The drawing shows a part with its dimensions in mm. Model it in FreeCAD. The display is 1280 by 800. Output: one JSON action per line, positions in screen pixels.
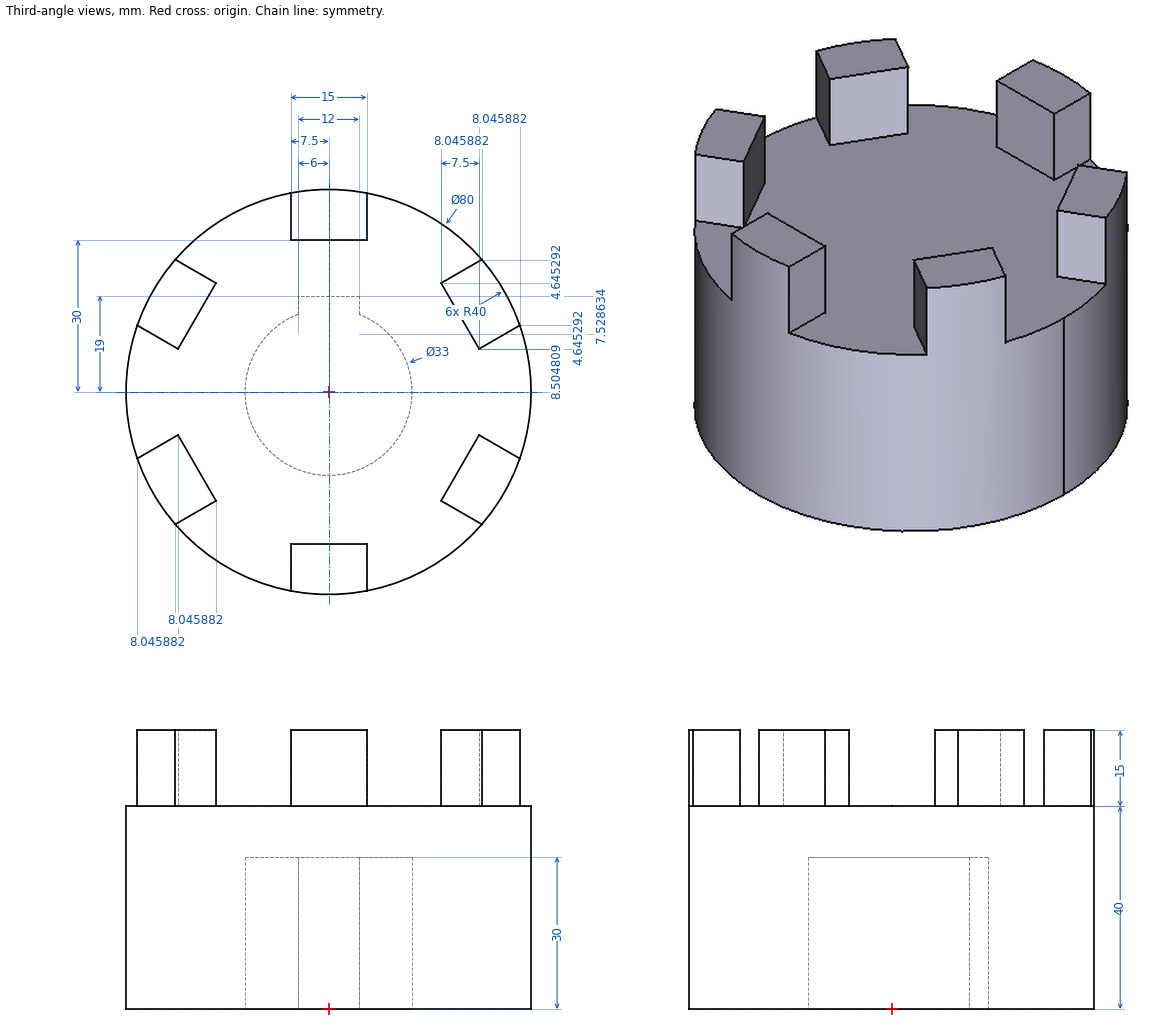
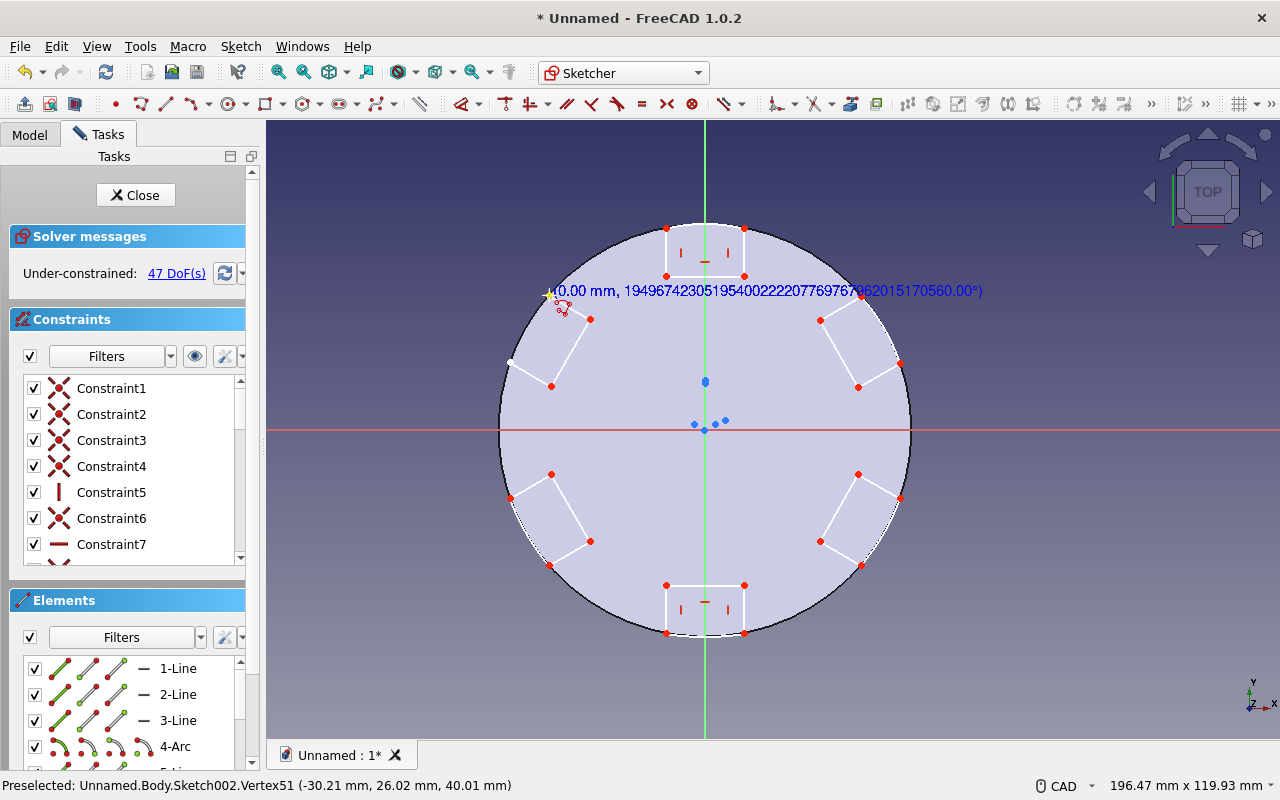
{"action": "key", "text": "g 3 a"}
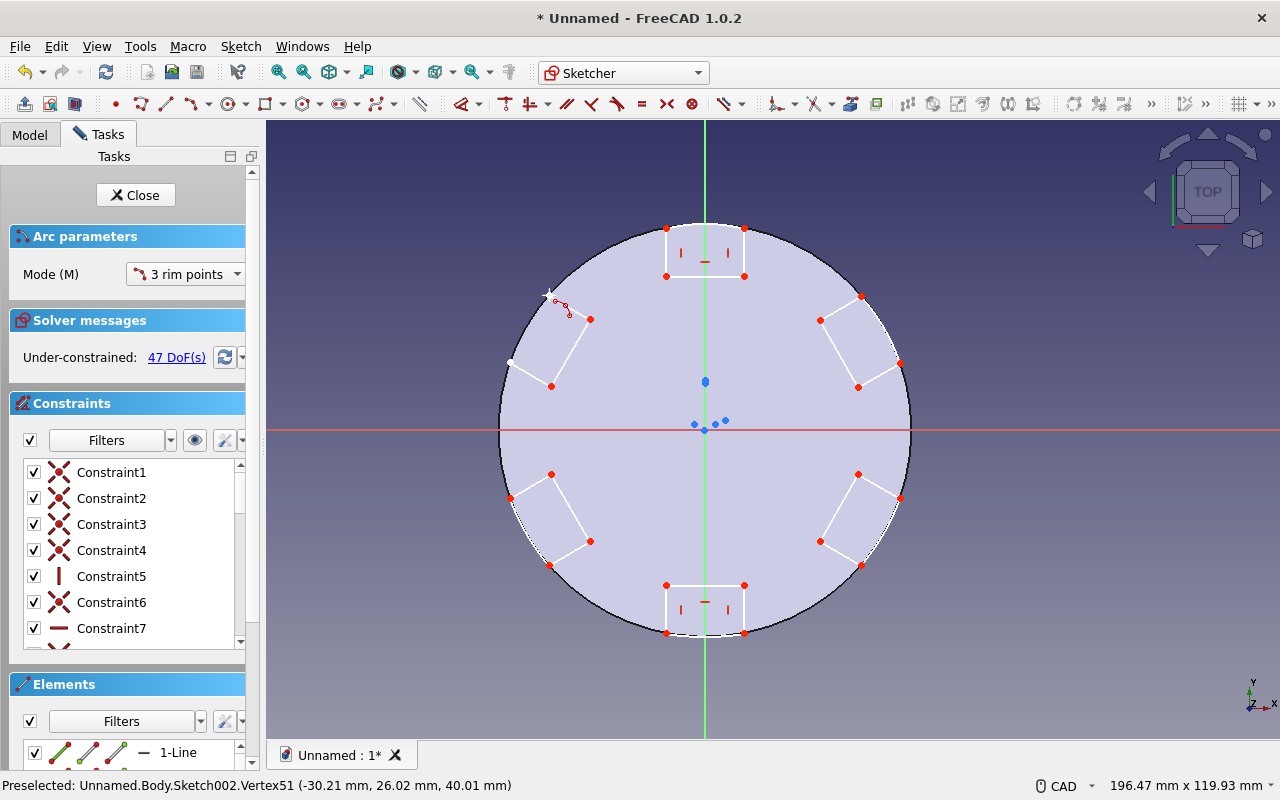
{"action": "left_click", "coordinate": [549, 296]}
{"action": "left_click", "coordinate": [510, 363]}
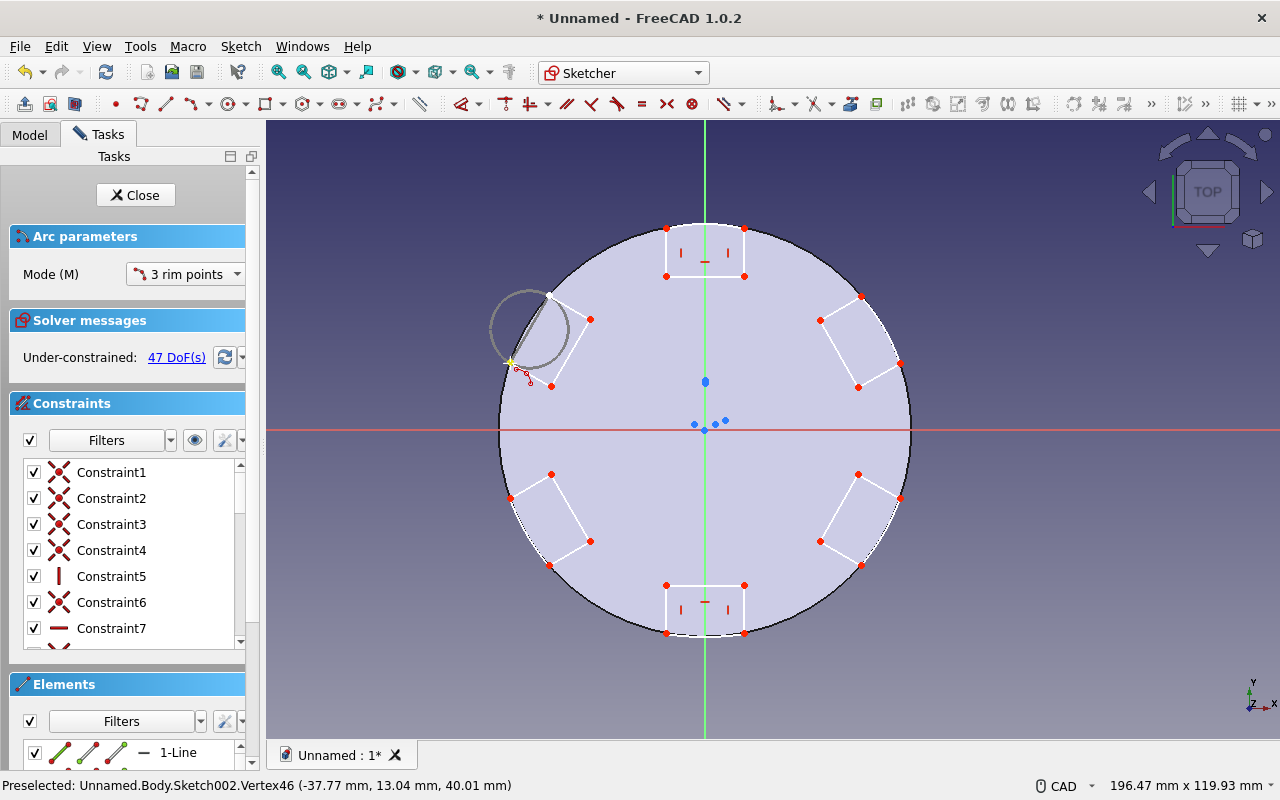
{"action": "scroll", "coordinate": [526, 327], "scroll_direction": "up", "scroll_amount": 8}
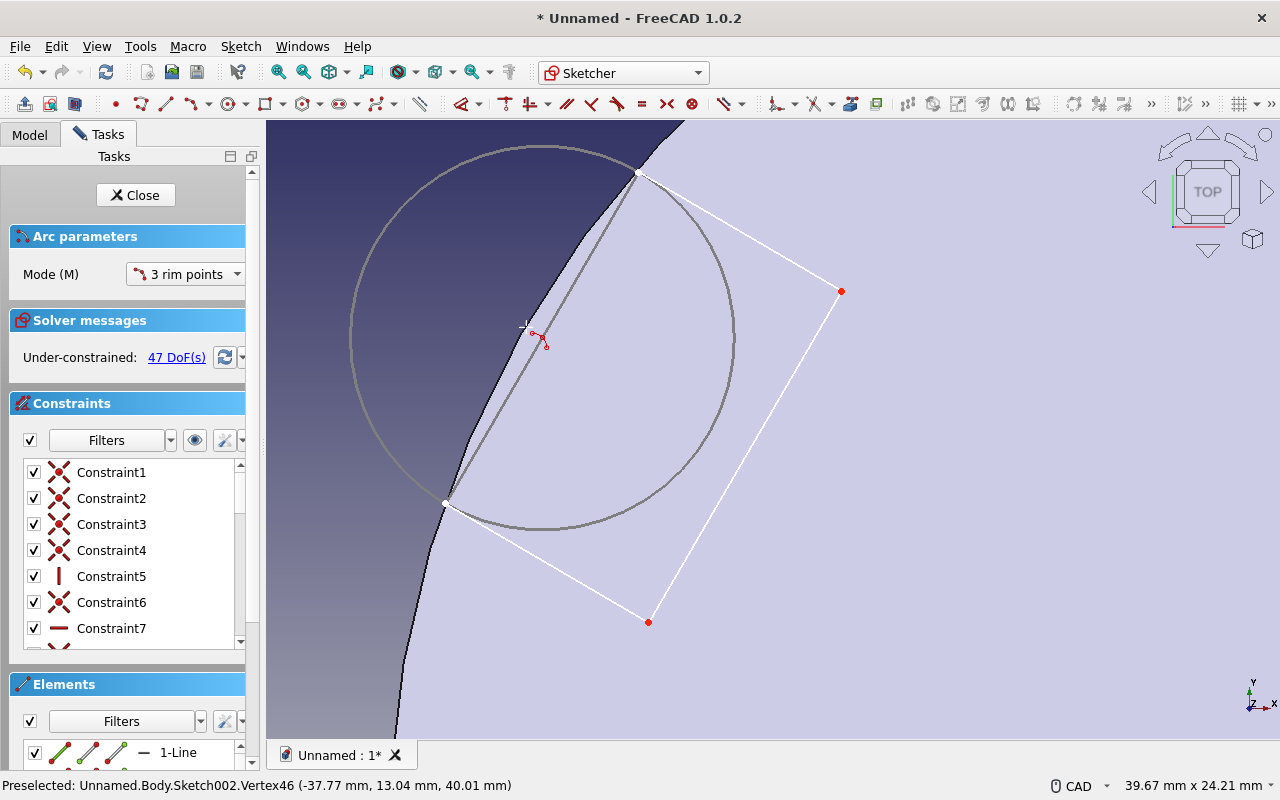
{"action": "left_click", "coordinate": [526, 326]}
{"action": "key", "text": "Escape"}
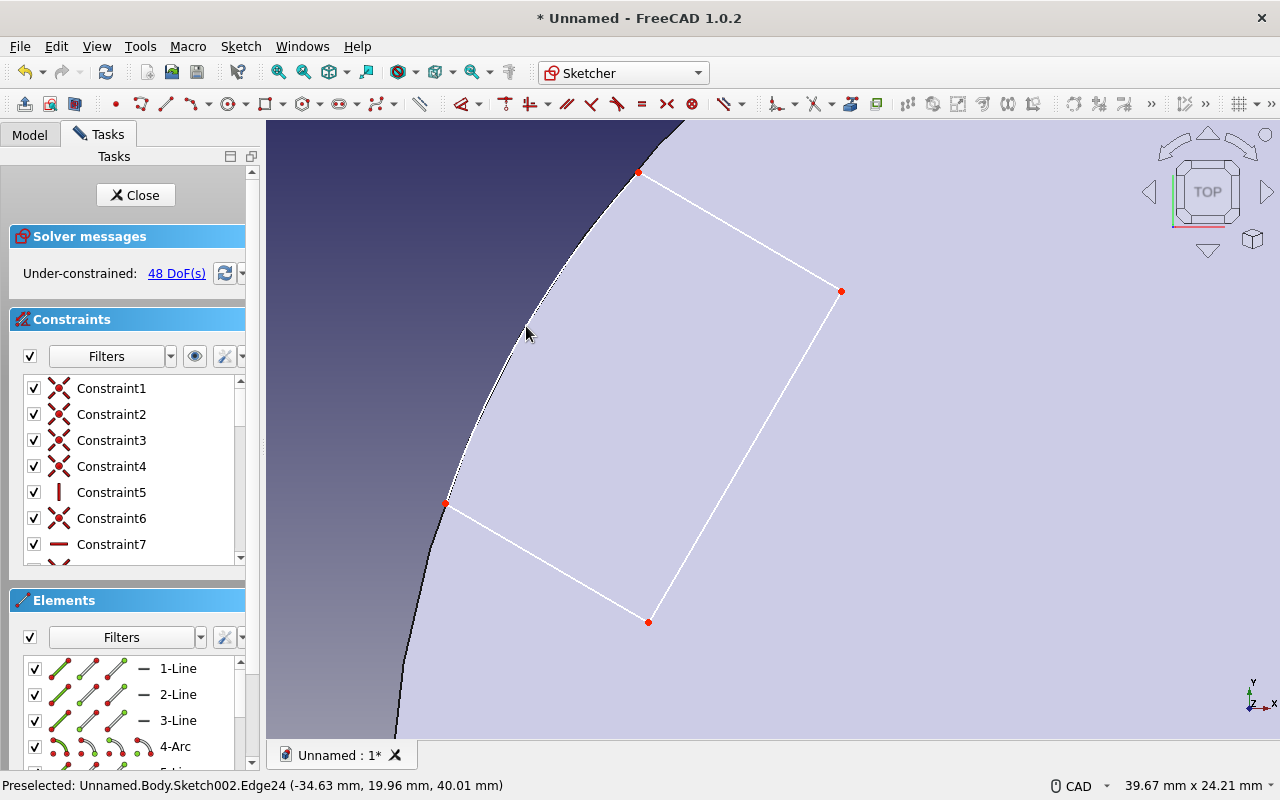
{"action": "scroll", "coordinate": [526, 326], "scroll_direction": "down", "scroll_amount": 8}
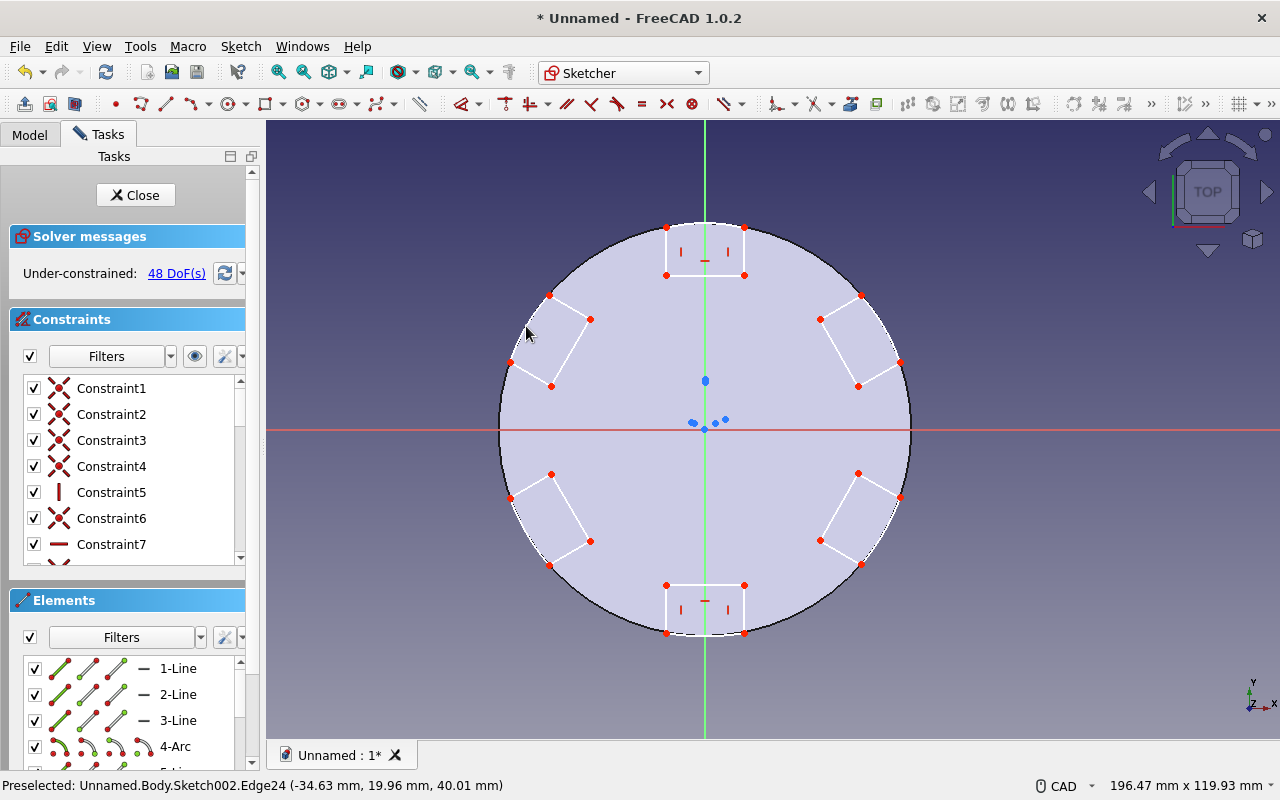
{"action": "left_click", "coordinate": [891, 341]}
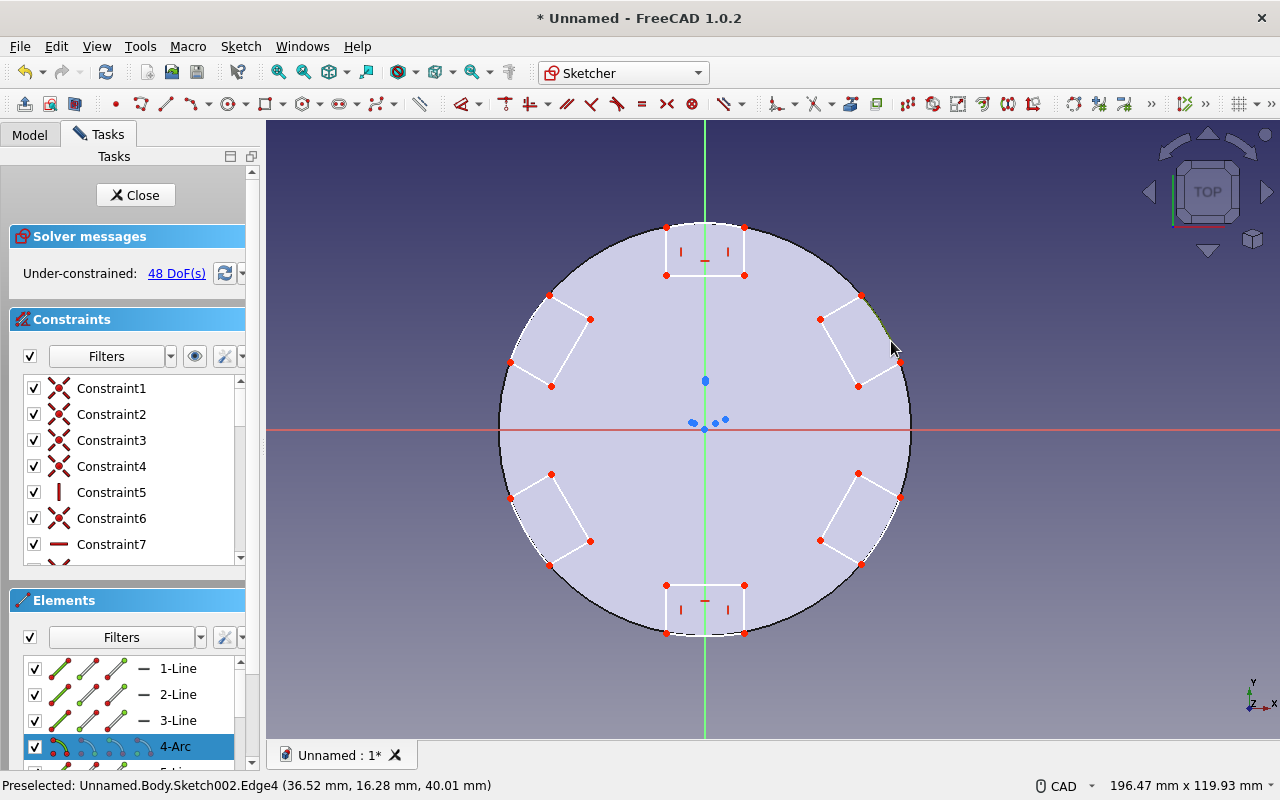
{"action": "left_click", "coordinate": [721, 224]}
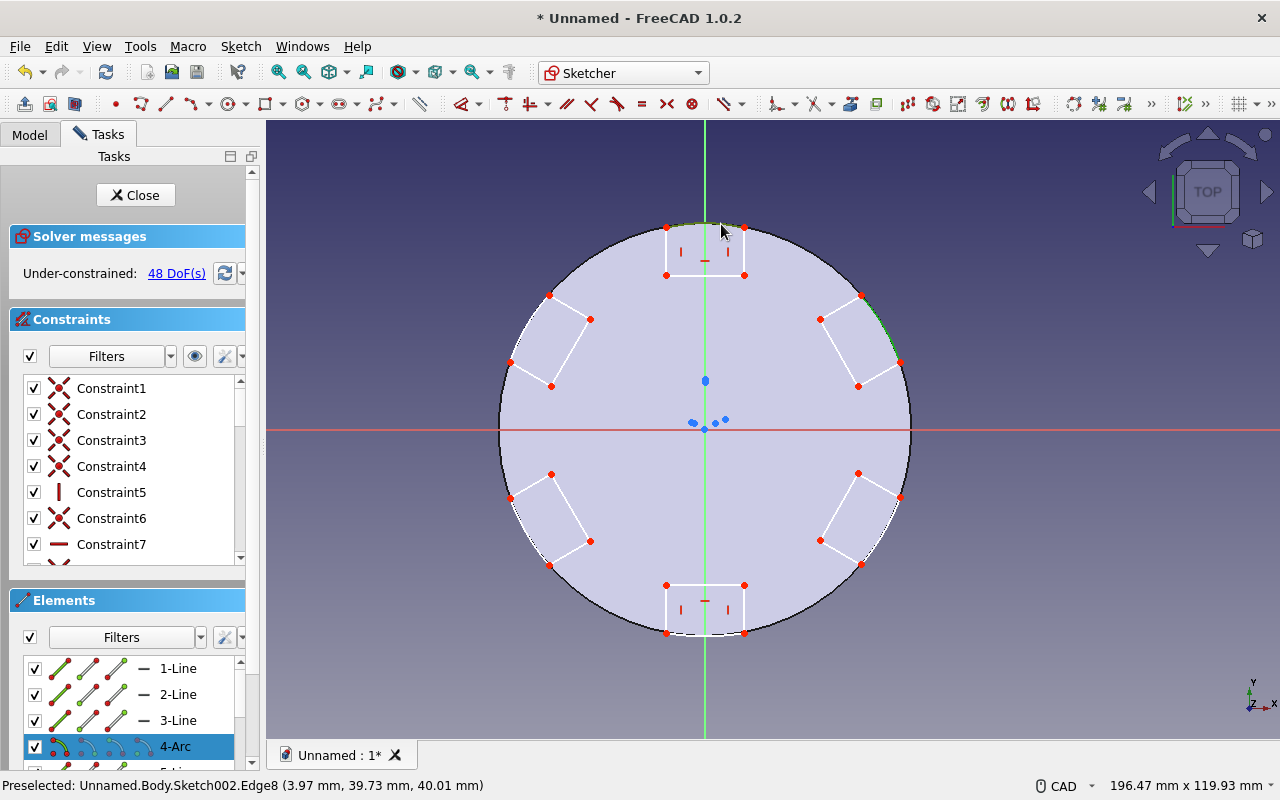
{"action": "key", "text": "c"}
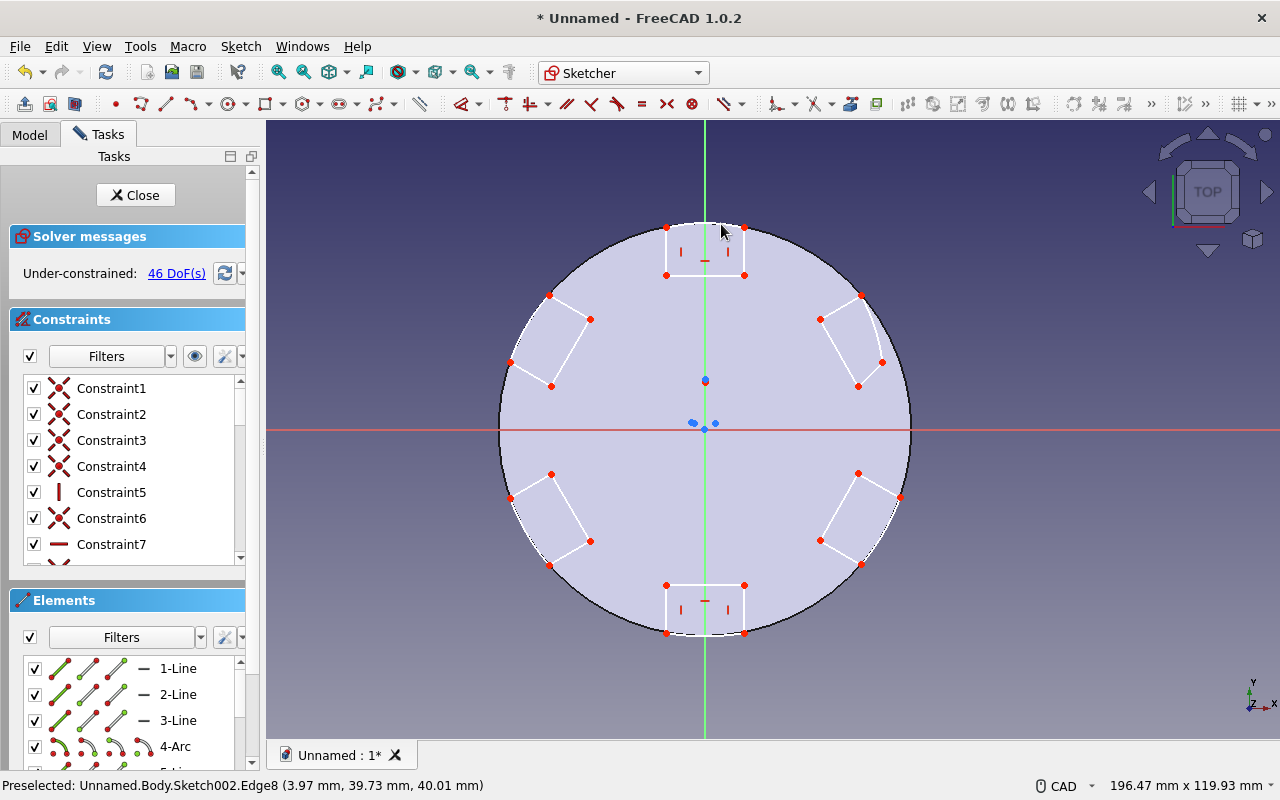
{"action": "left_click", "coordinate": [879, 342]}